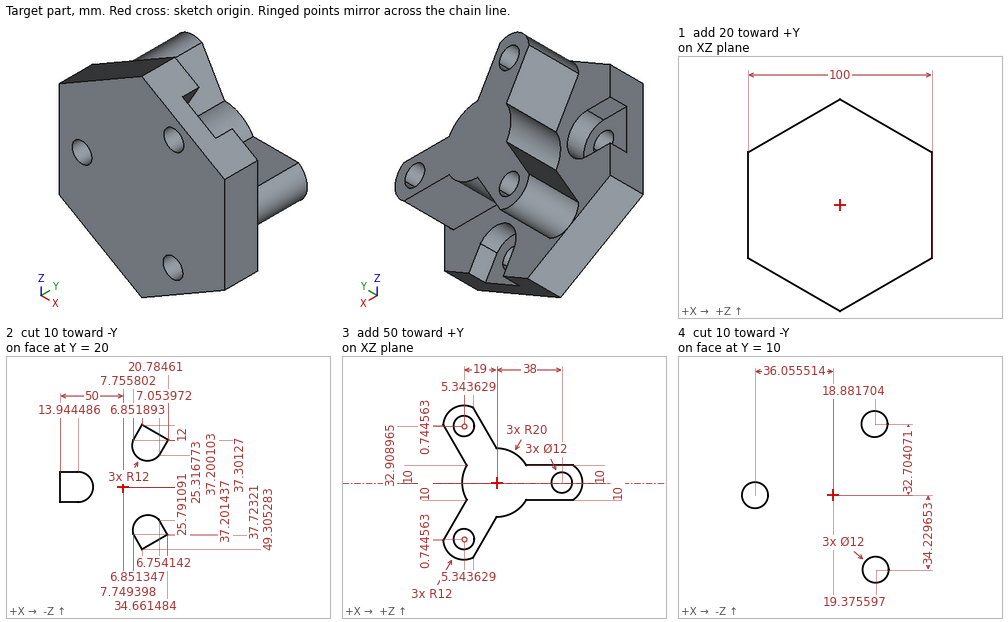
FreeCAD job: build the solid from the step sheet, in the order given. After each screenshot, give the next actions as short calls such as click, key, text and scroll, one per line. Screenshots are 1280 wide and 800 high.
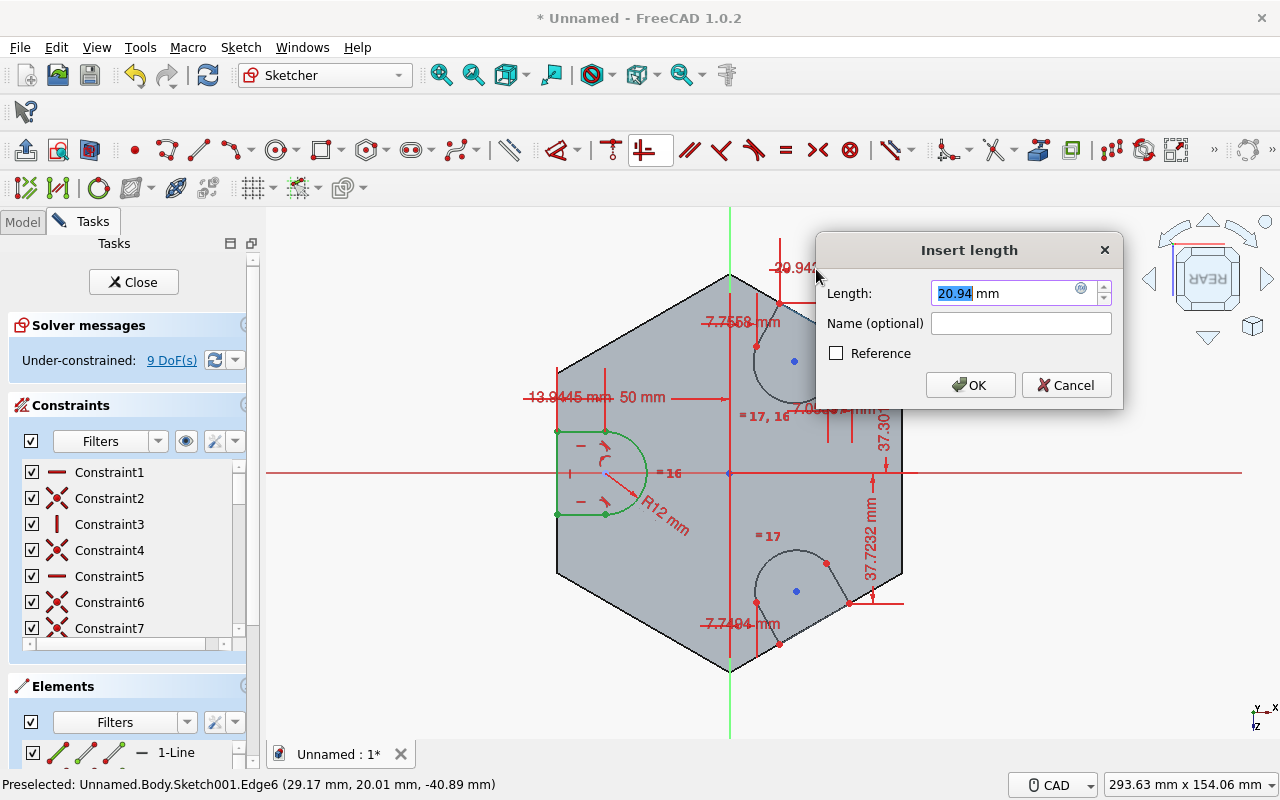
text(20.78461)
key(Return)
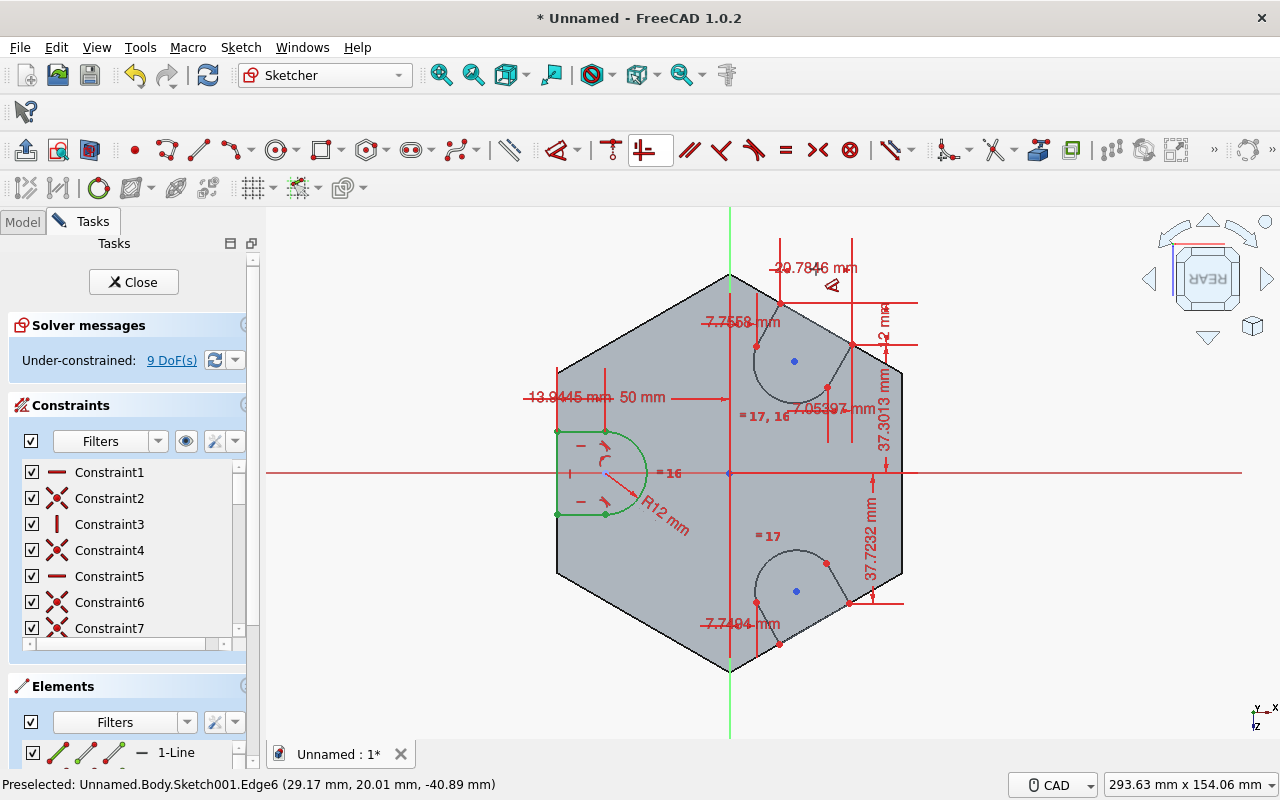
scroll(773, 316, up, 3)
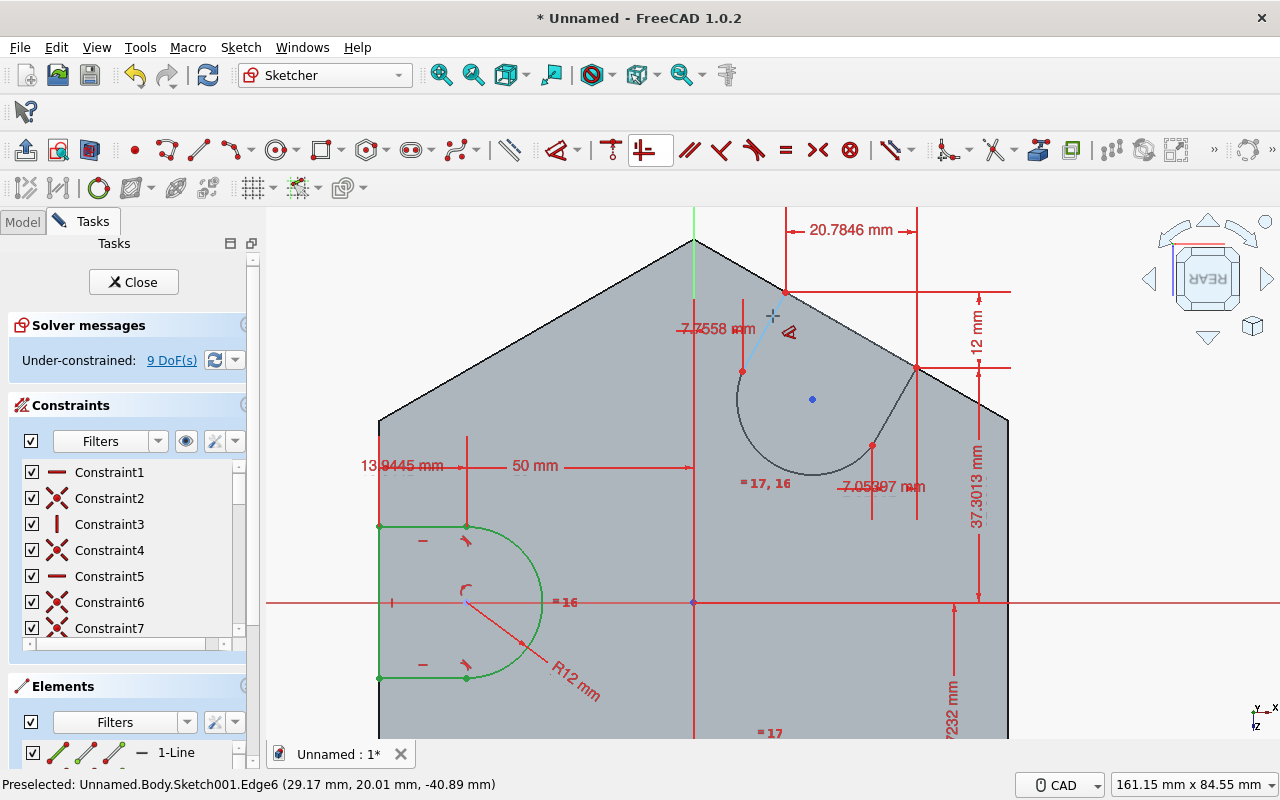
click(773, 316)
click(764, 258)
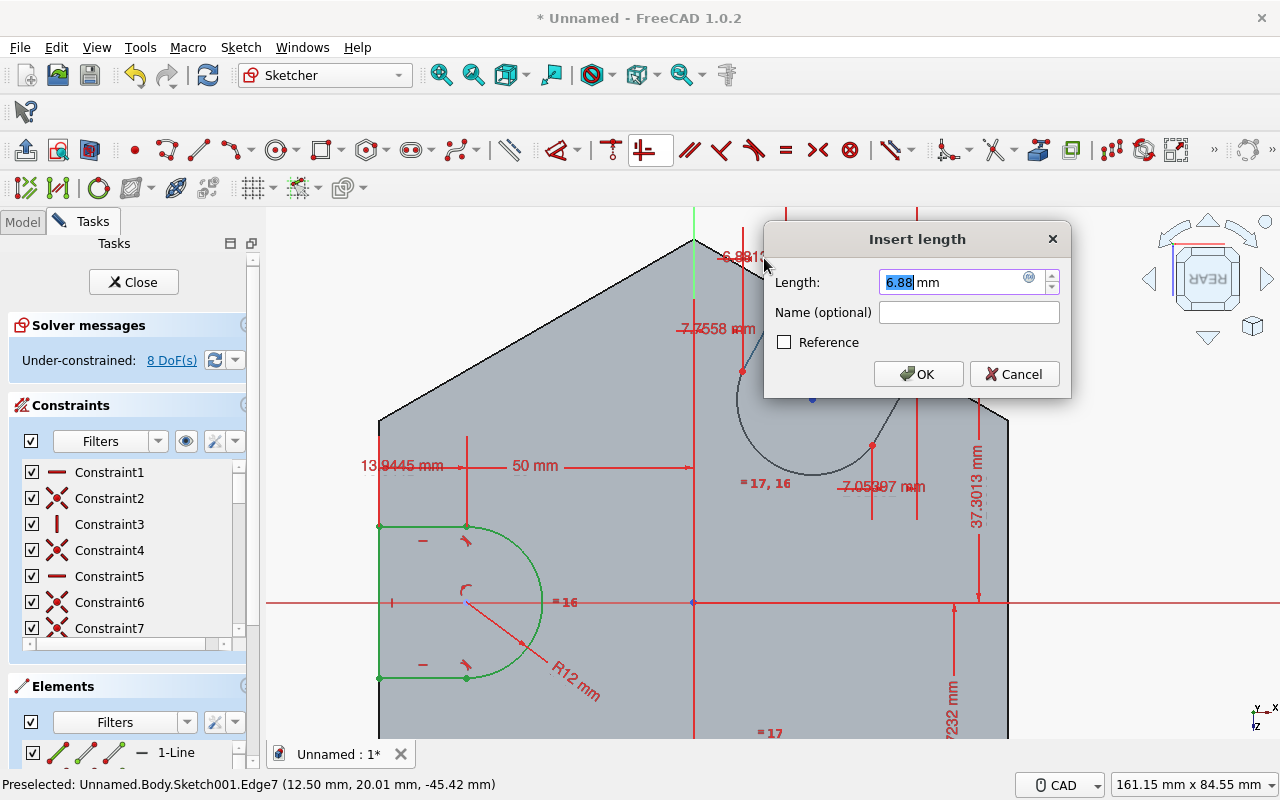
text(6.851893)
key(Return)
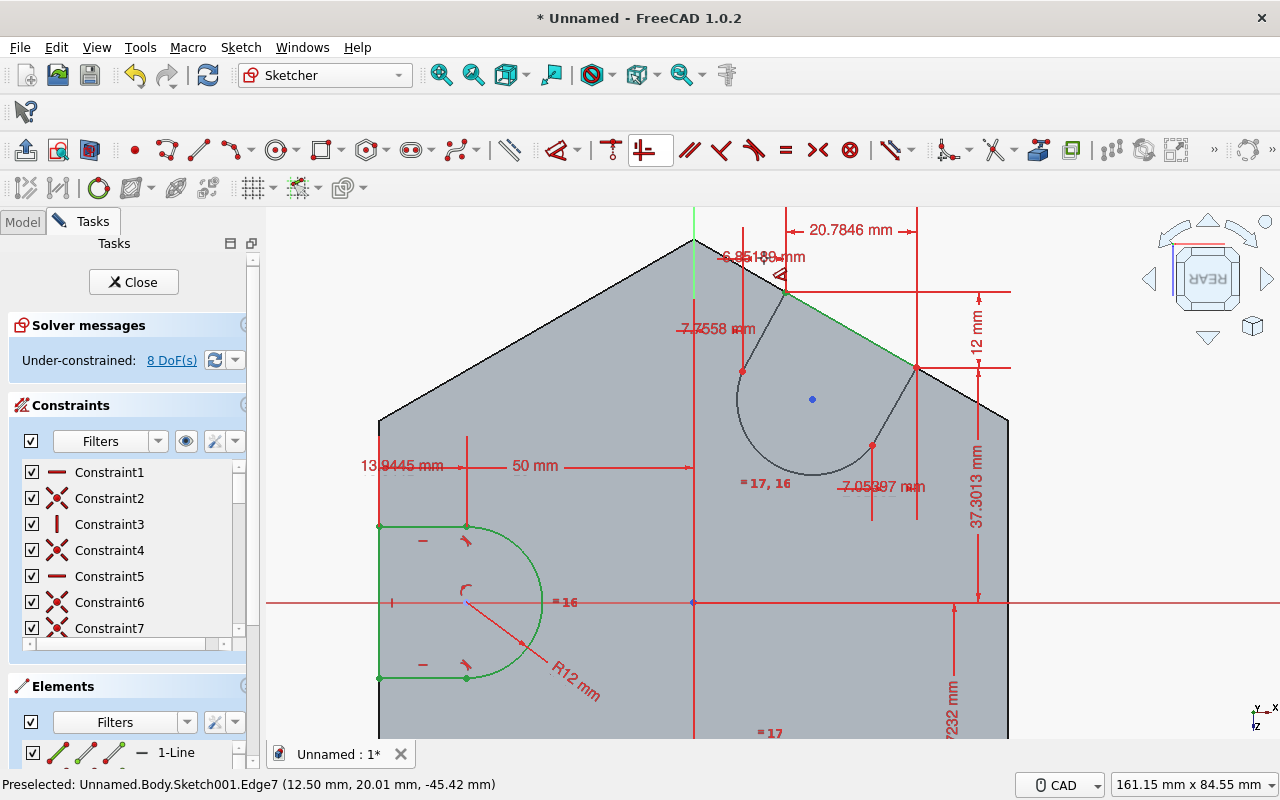
scroll(773, 315, down, 3)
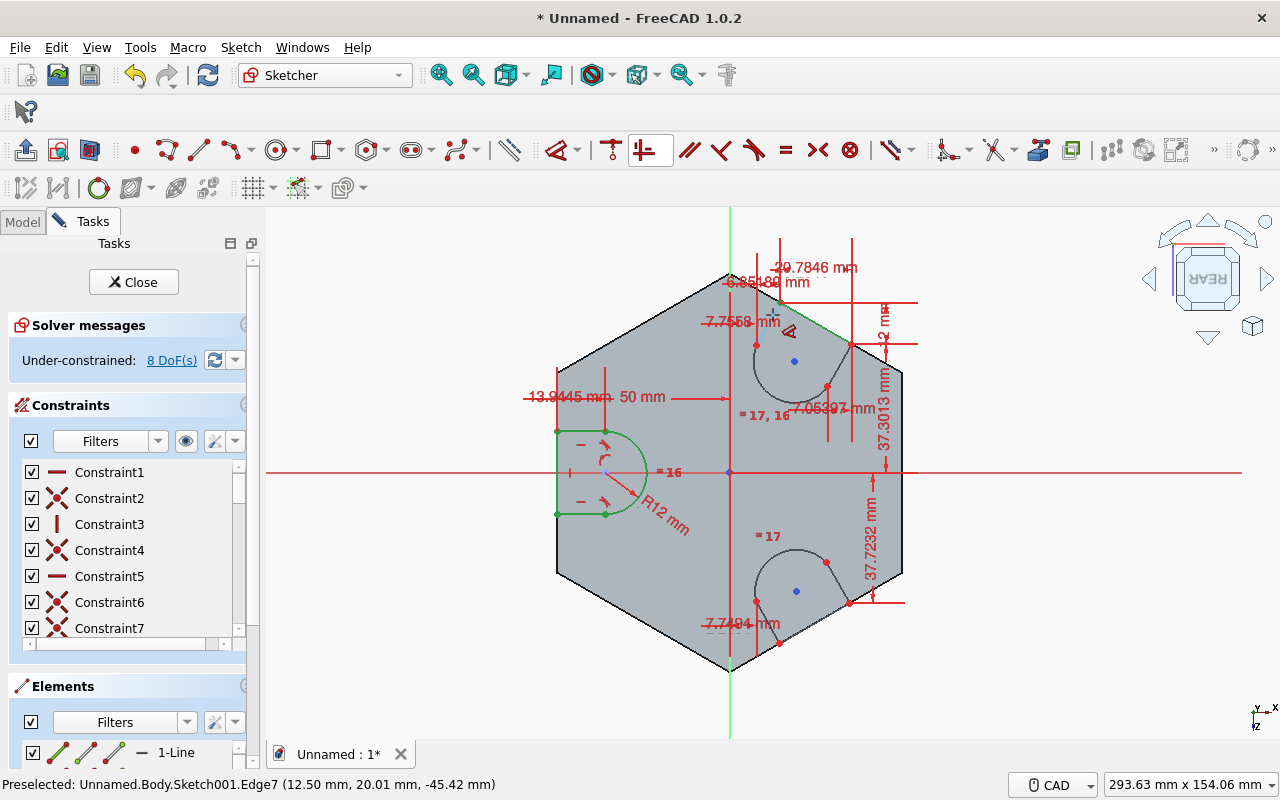
scroll(764, 614, up, 3)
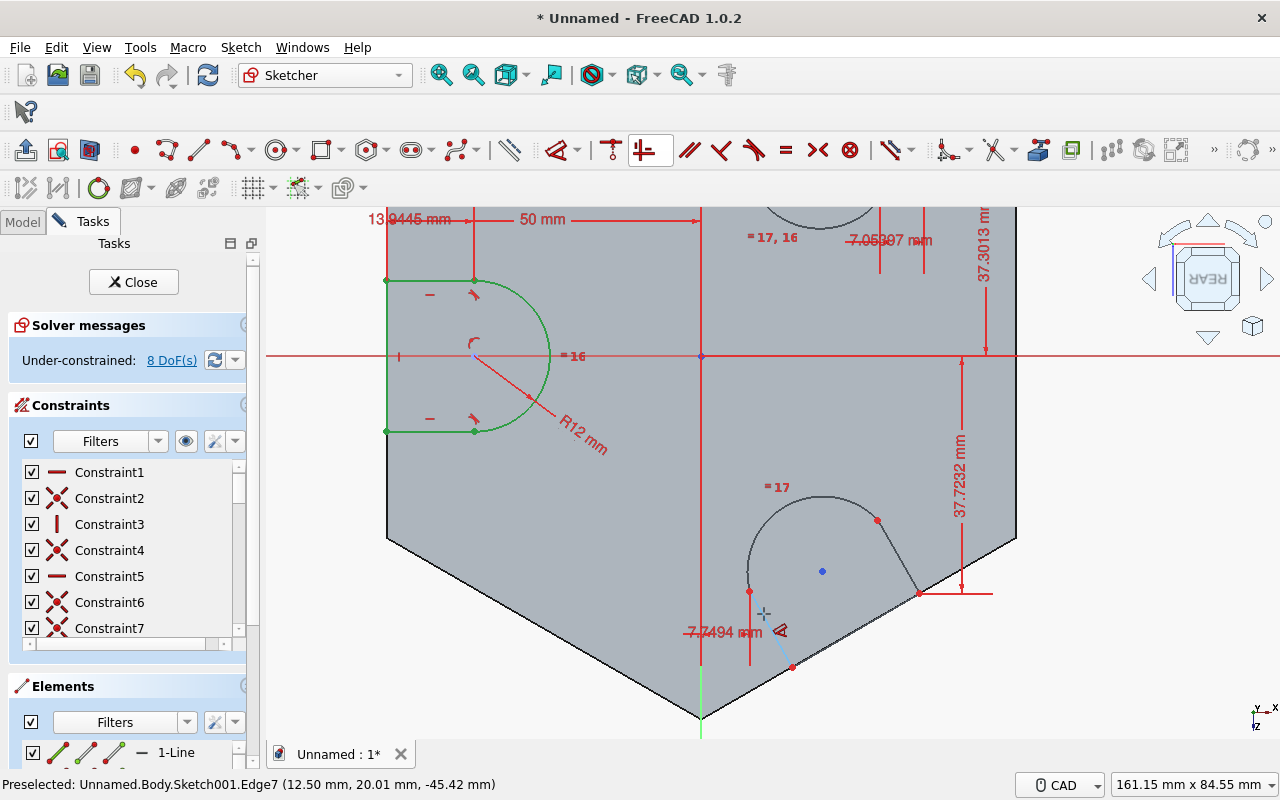
click(763, 614)
click(771, 702)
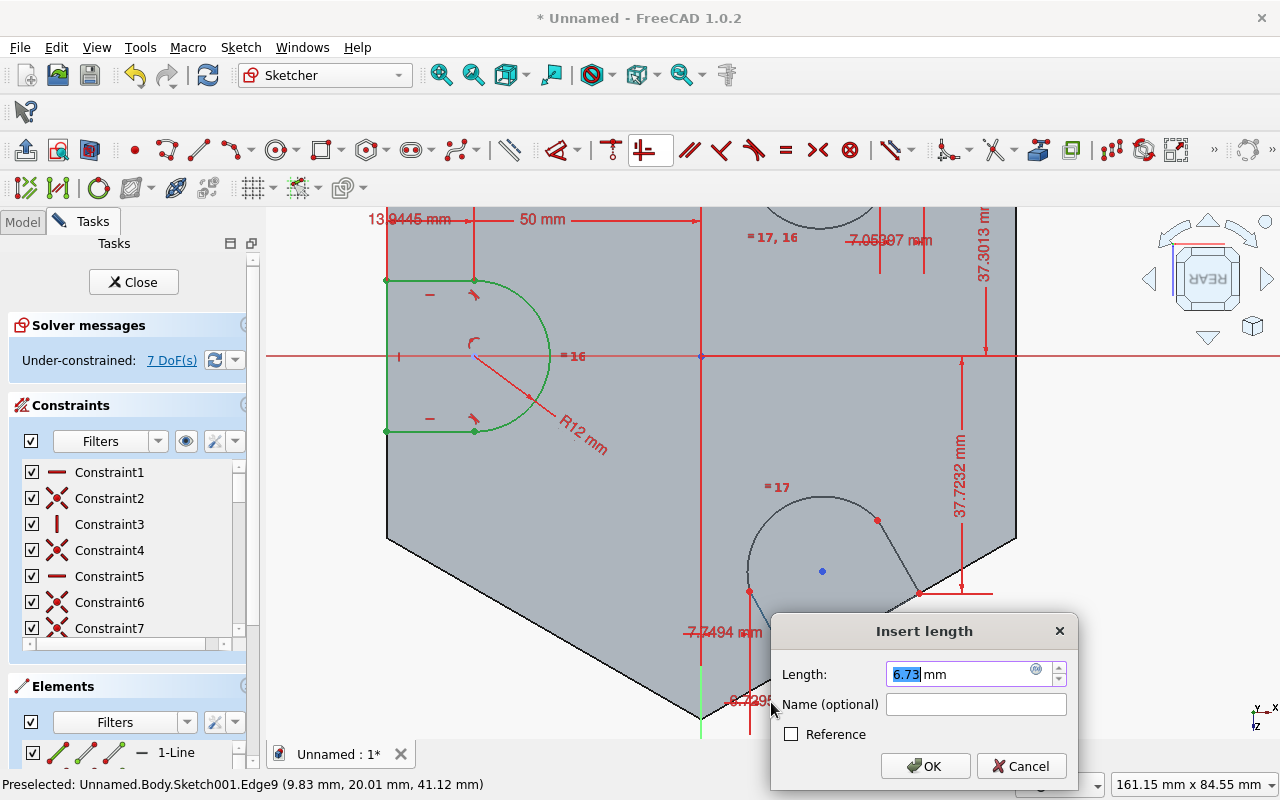
text(6.851347)
key(Return)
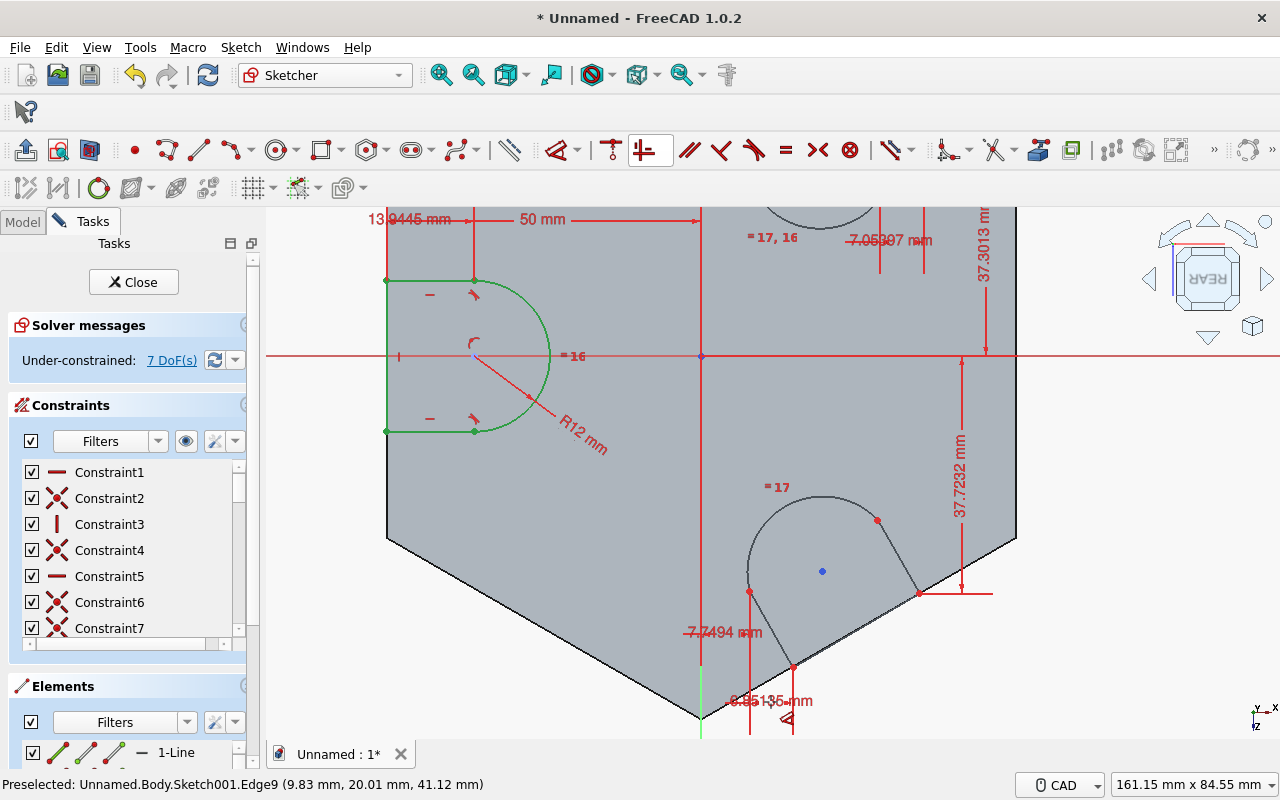
click(907, 572)
click(899, 628)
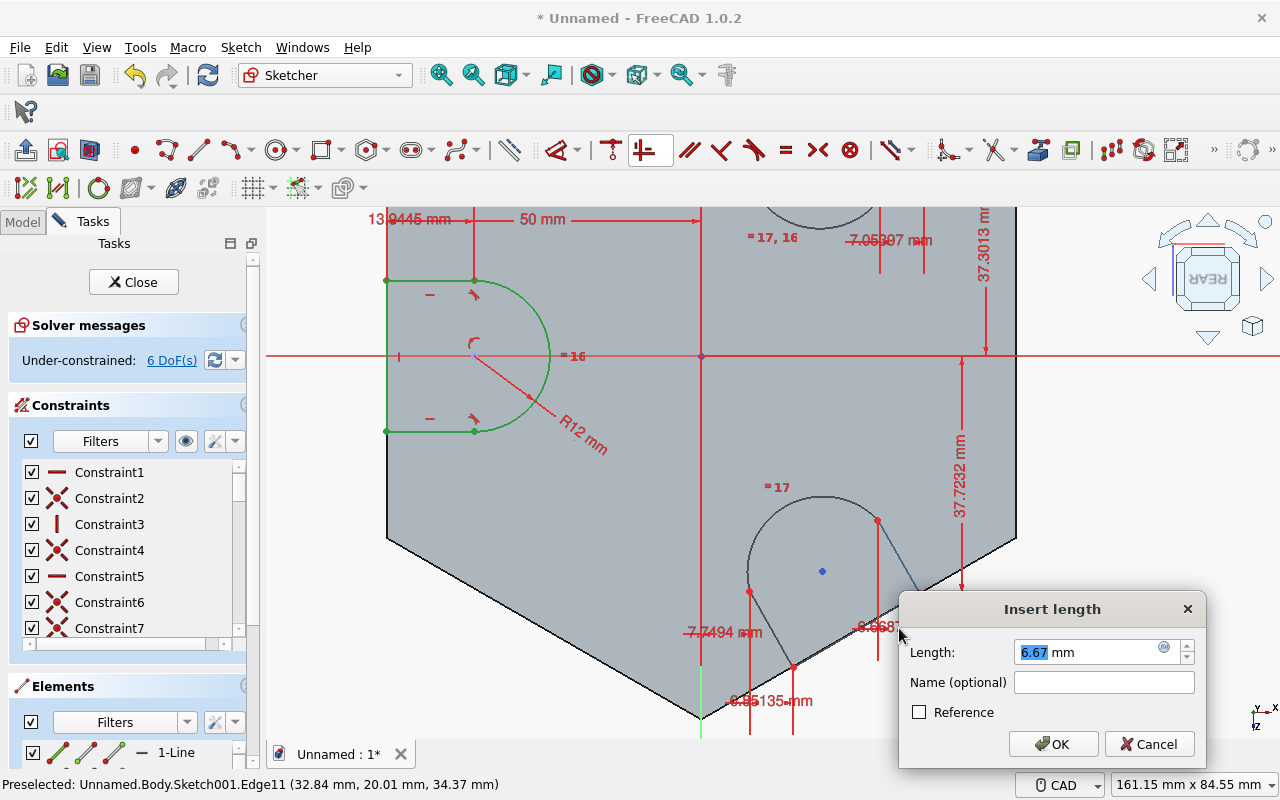
text(6.754142)
key(Return)